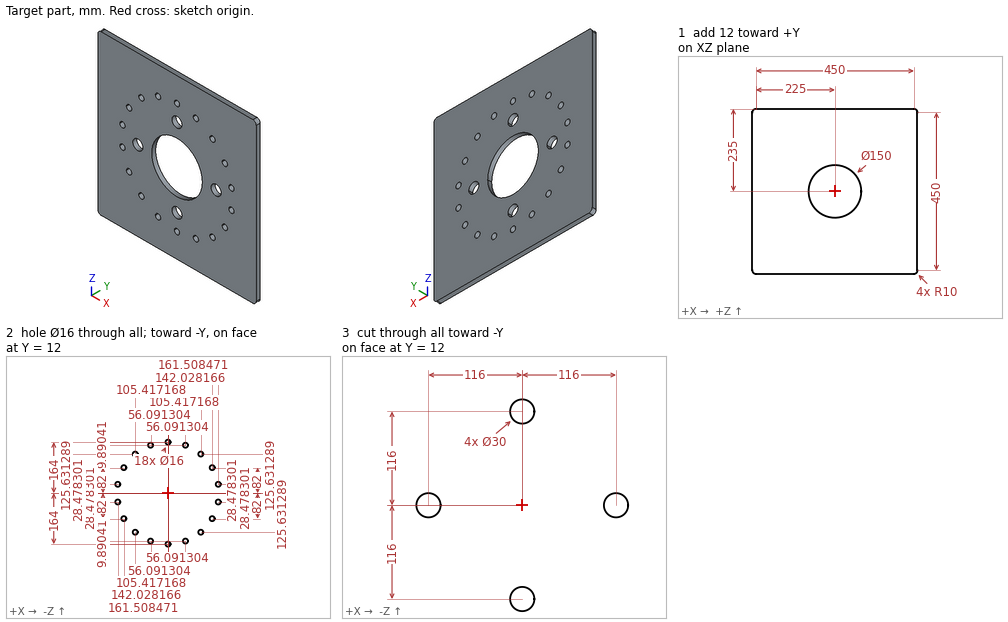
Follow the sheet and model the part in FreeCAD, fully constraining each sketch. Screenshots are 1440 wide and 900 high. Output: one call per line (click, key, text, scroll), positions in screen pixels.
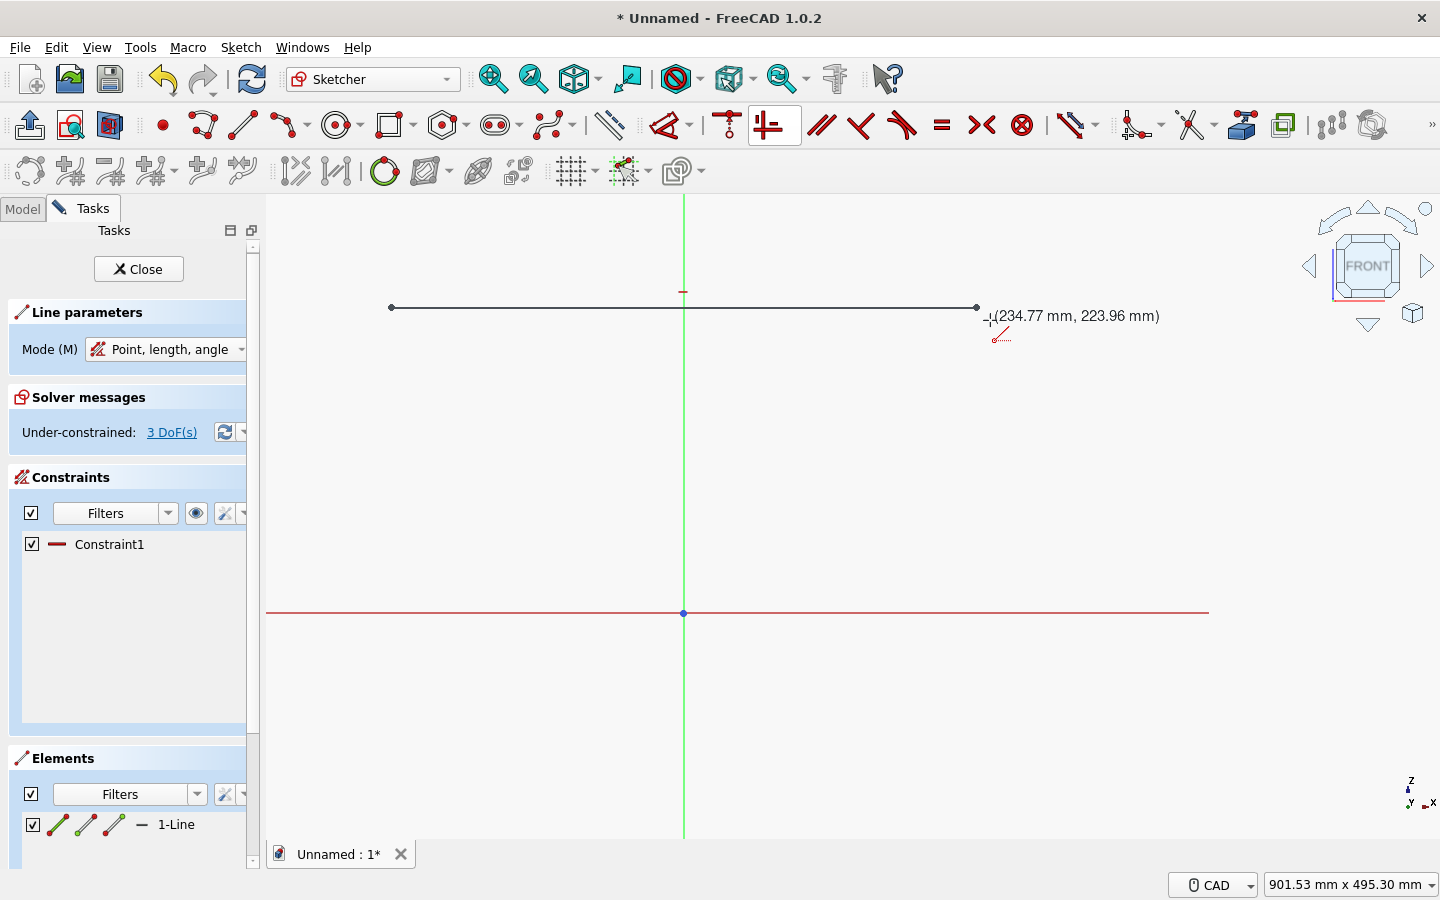
click(990, 320)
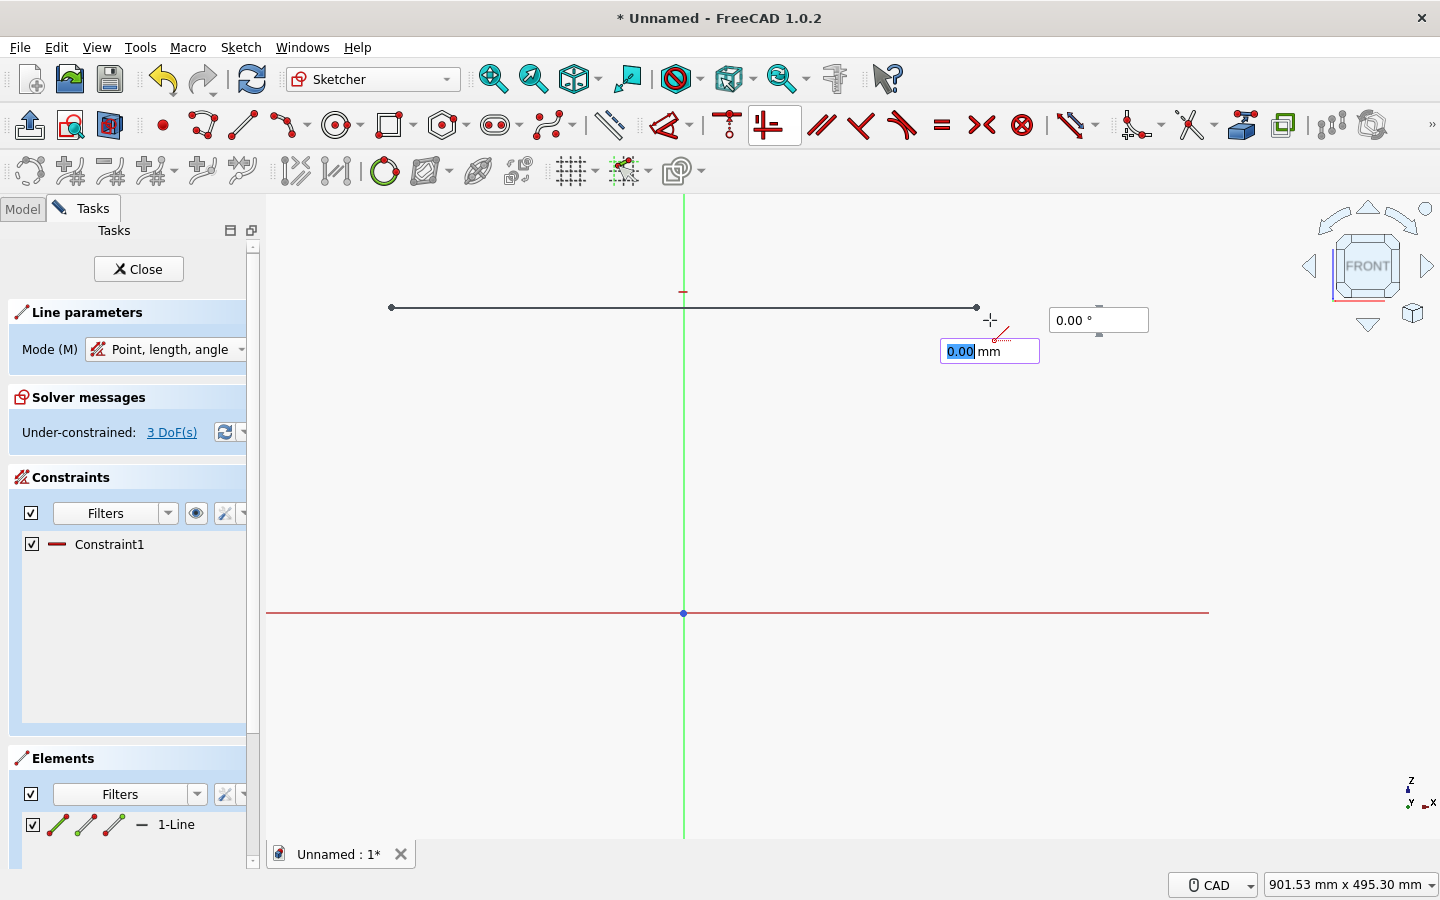
scroll(989, 320, down, 2)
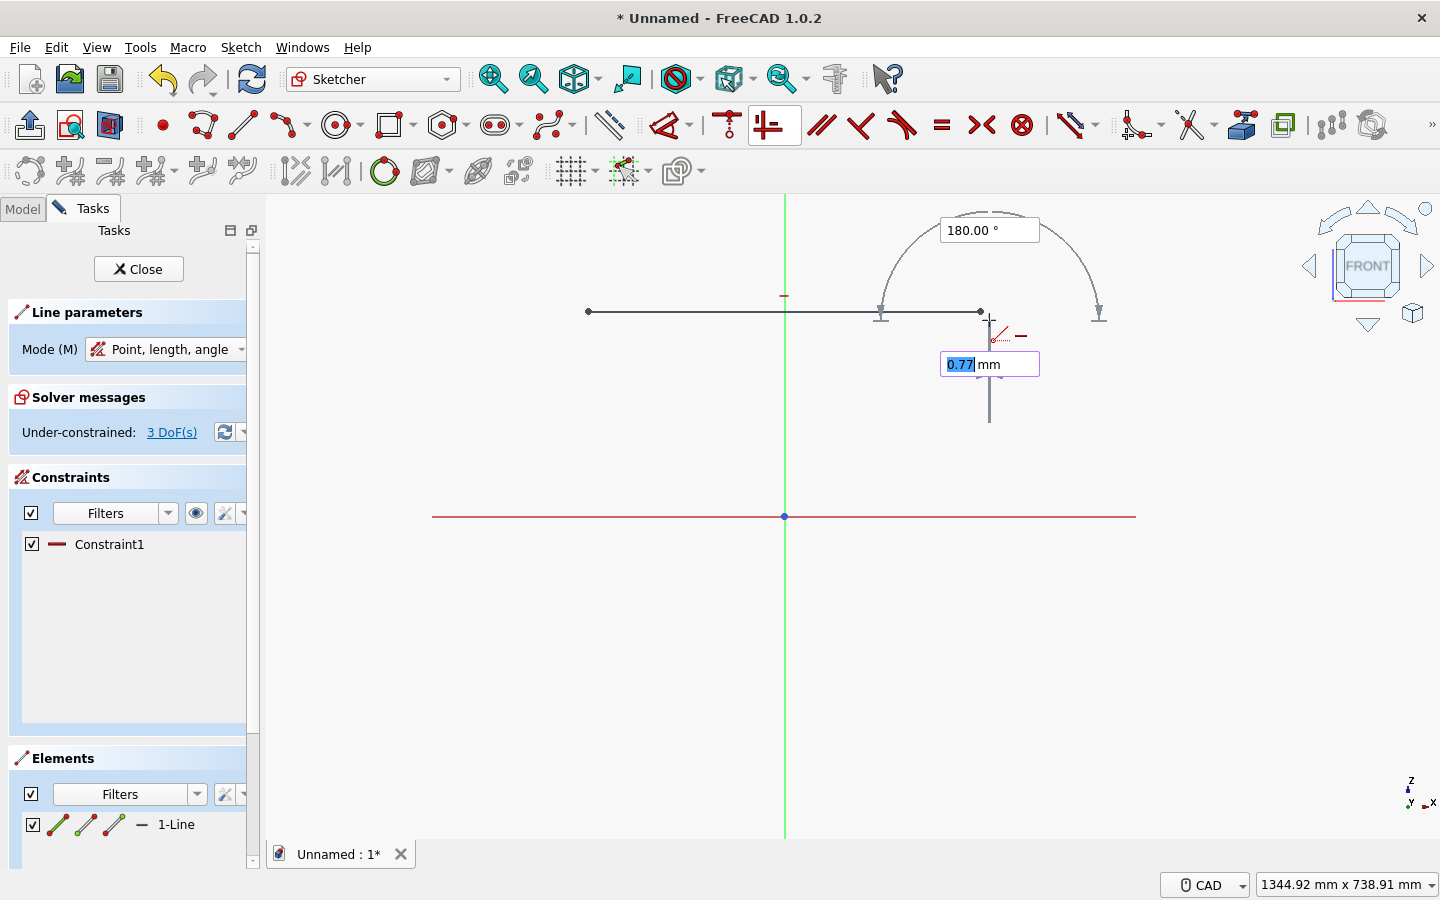
click(990, 713)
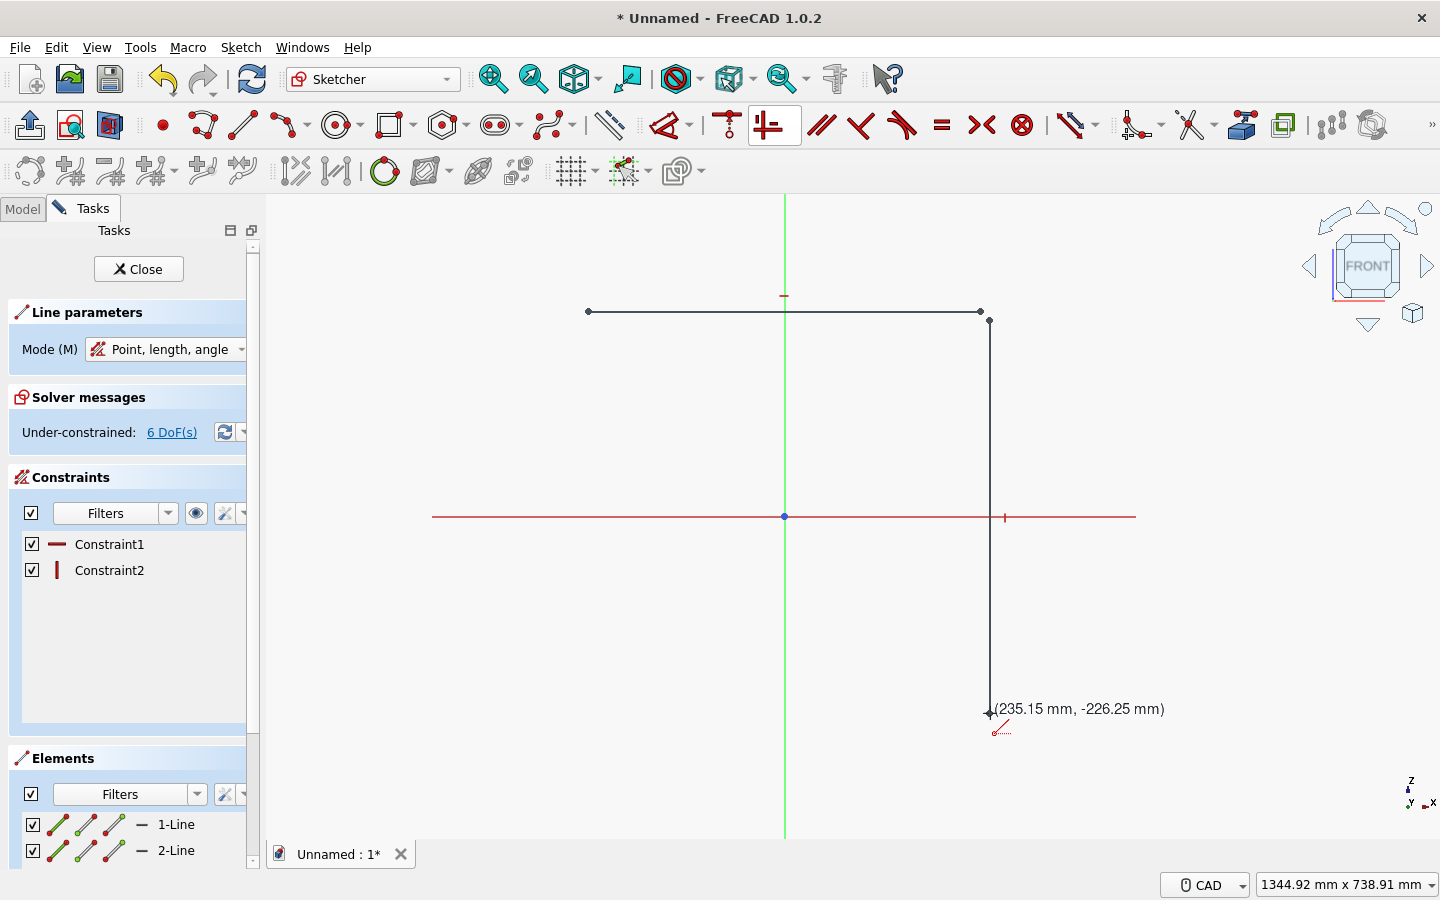
scroll(981, 722, up, 2)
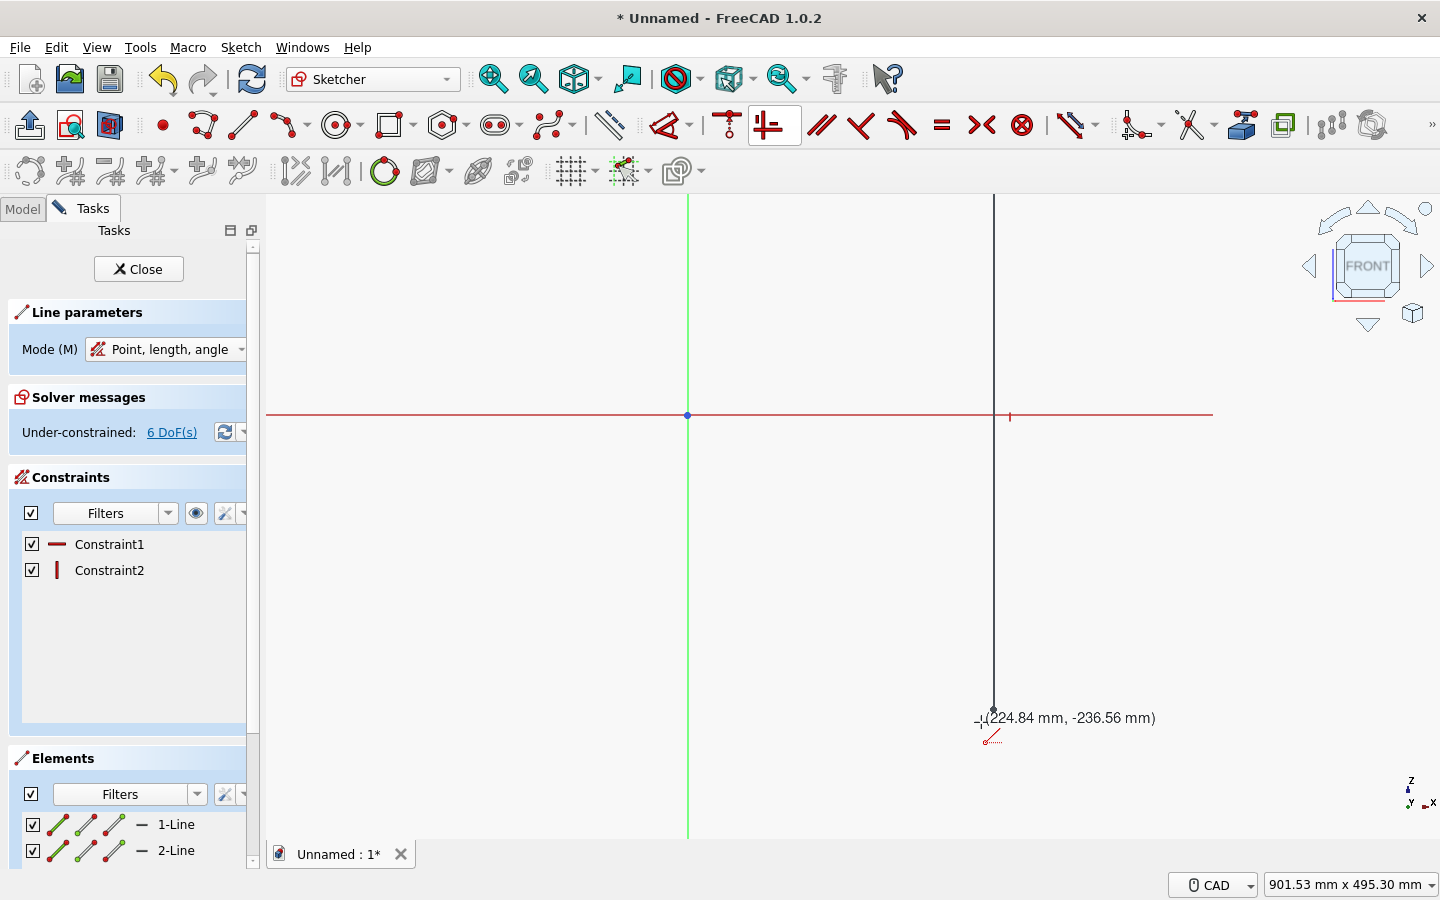
click(981, 721)
click(395, 721)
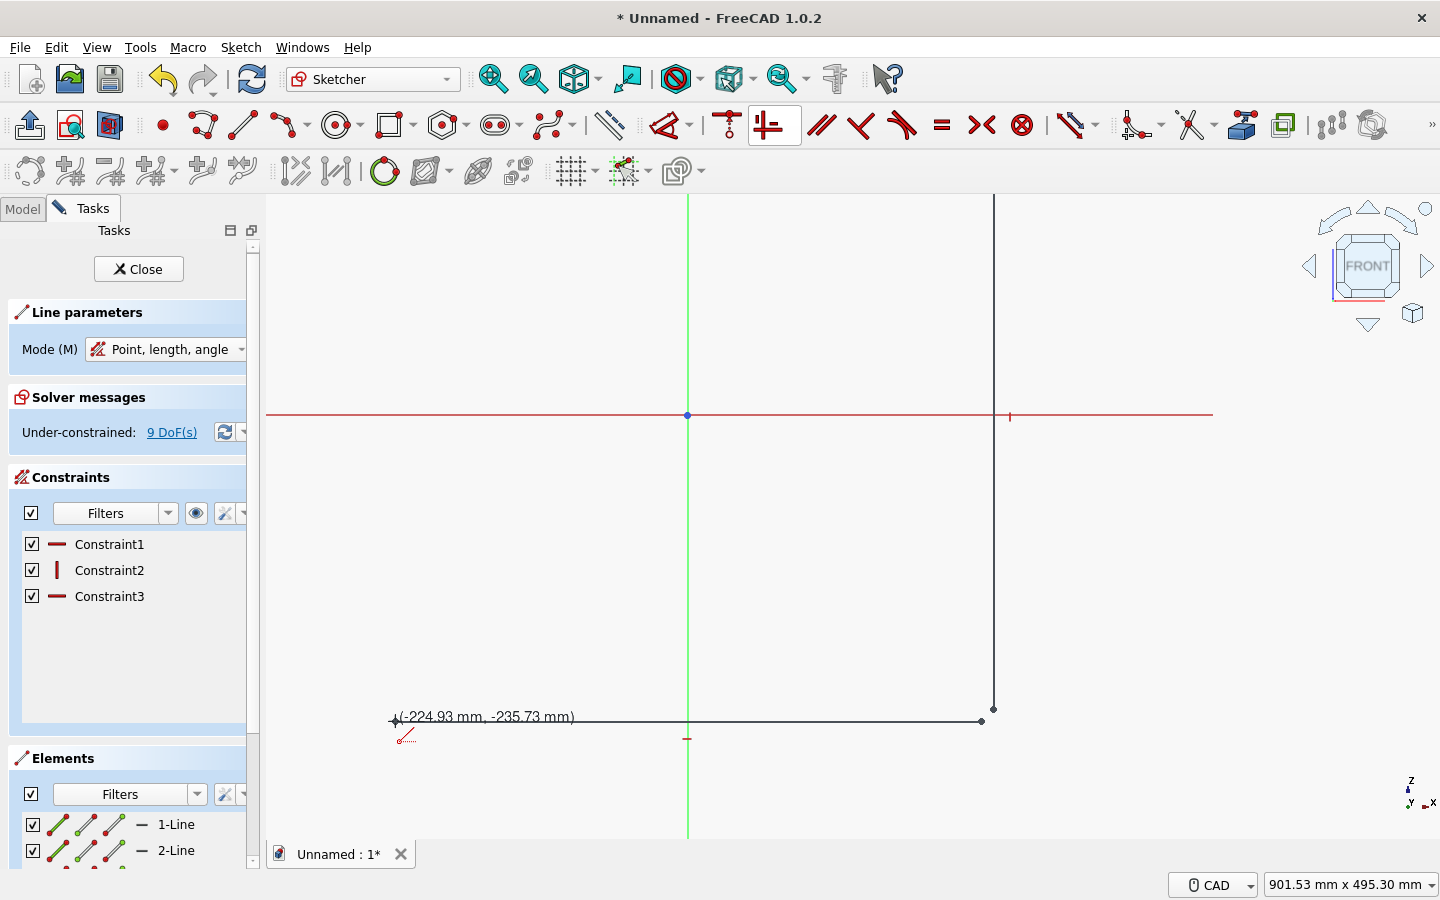
click(382, 708)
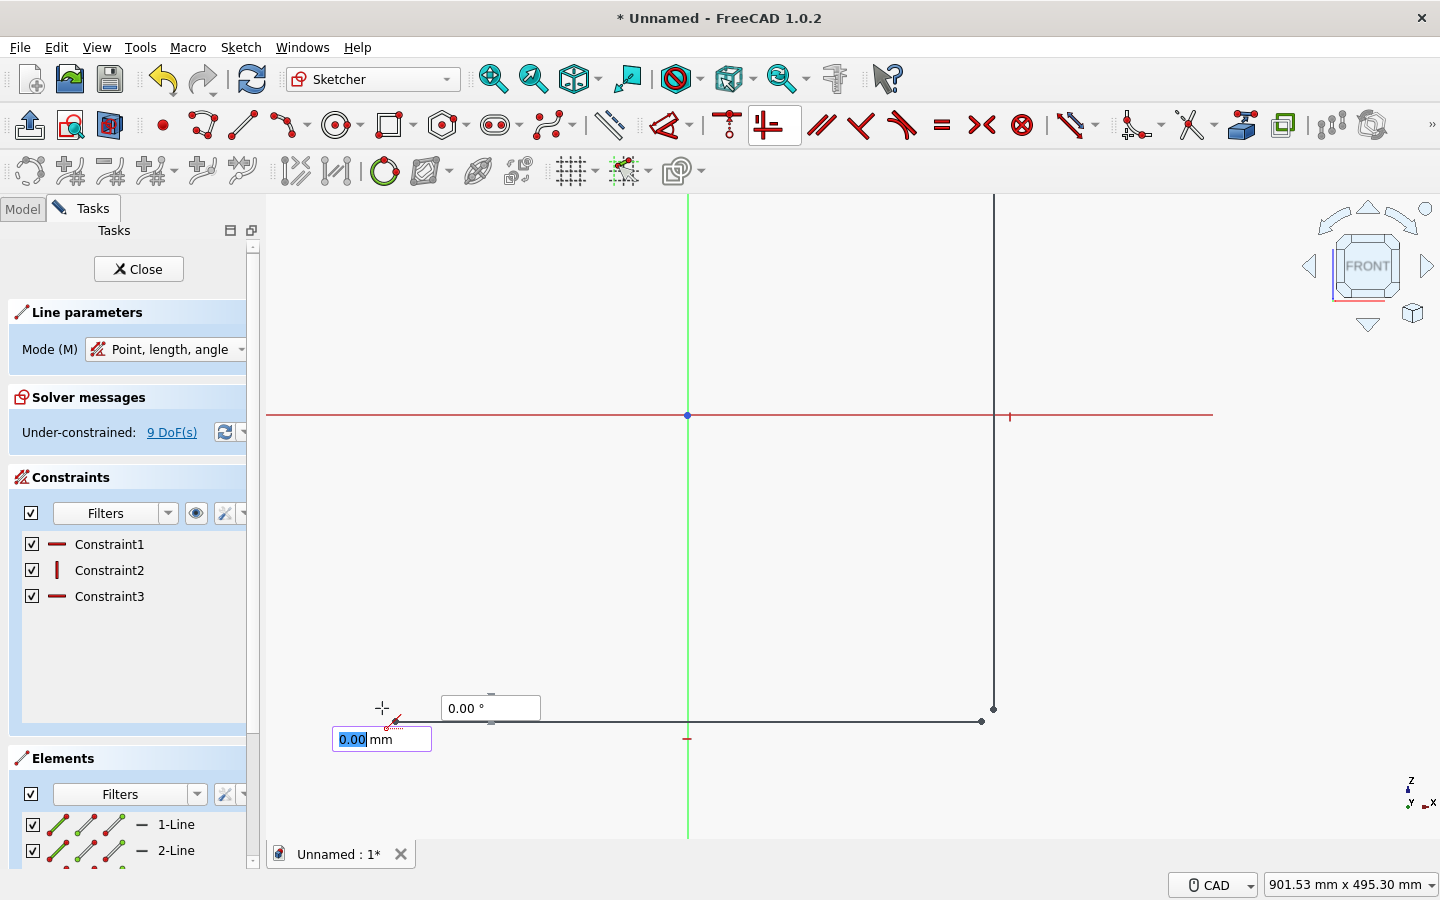
scroll(981, 723, down, 2)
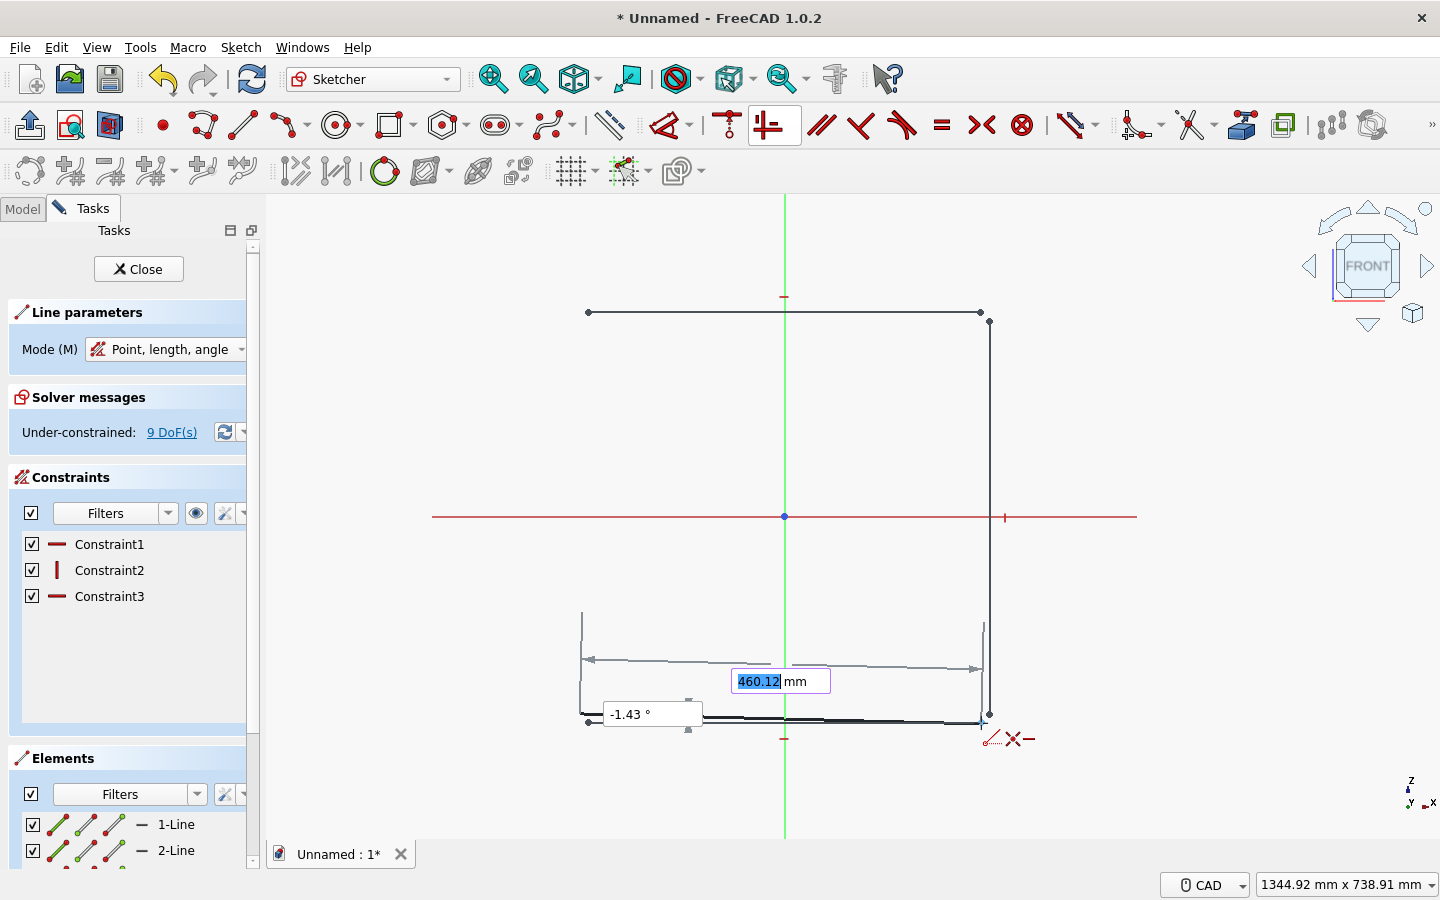
scroll(580, 320, up, 2)